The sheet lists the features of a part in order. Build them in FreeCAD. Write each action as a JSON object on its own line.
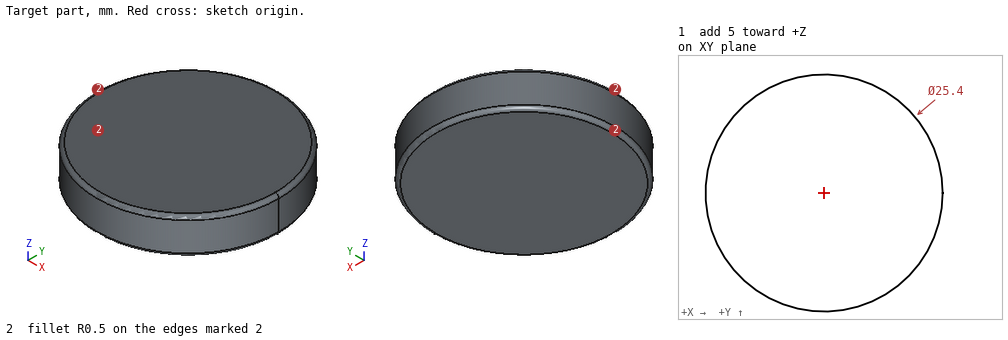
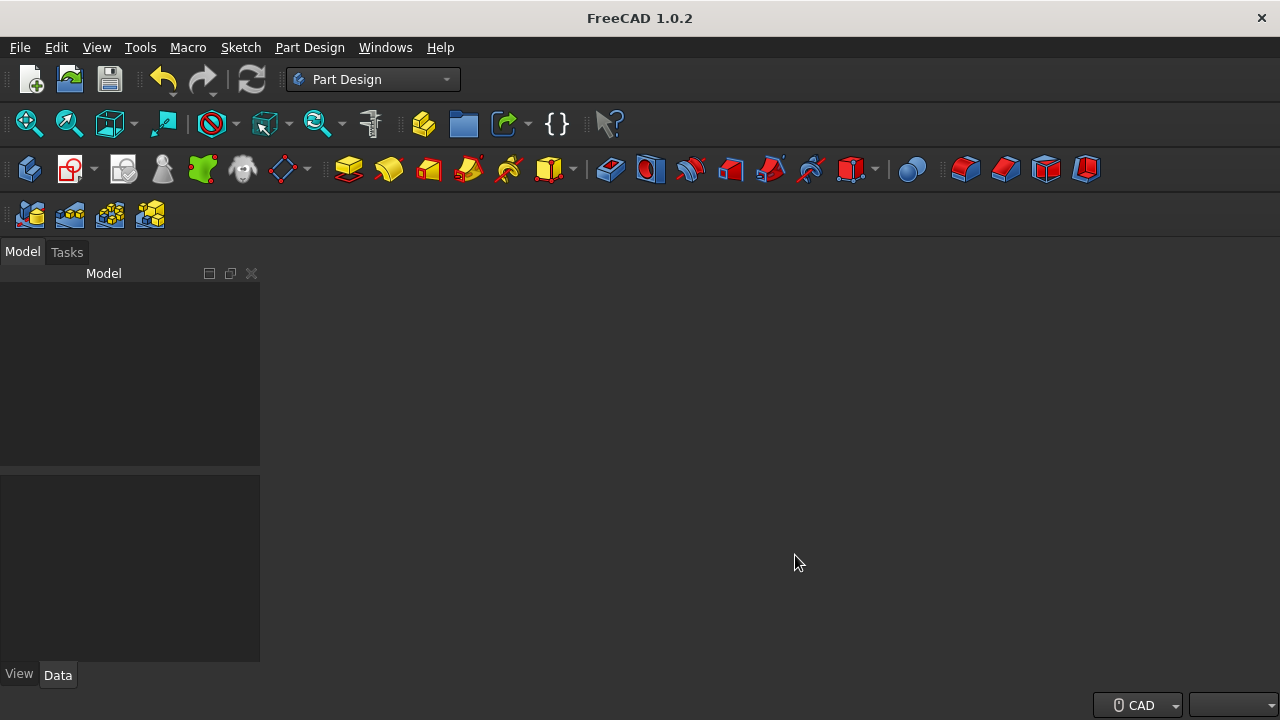
{"action": "left_click", "coordinate": [30, 80]}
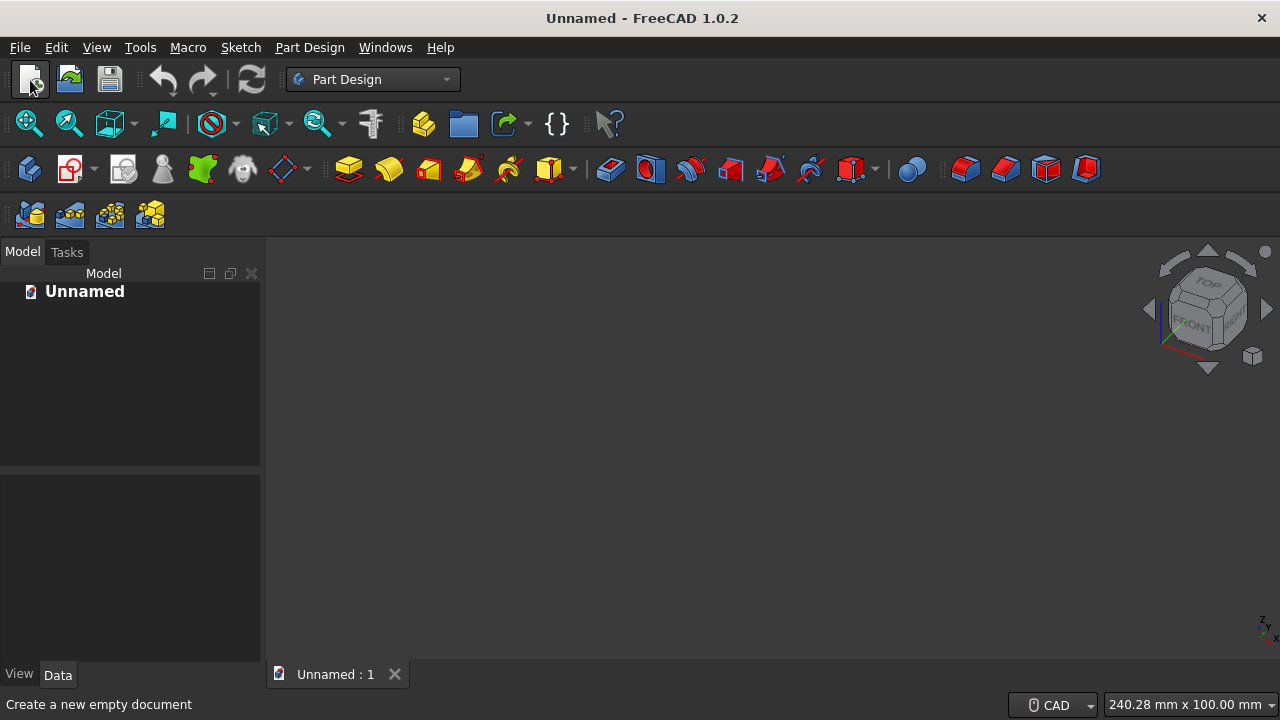
{"action": "left_click", "coordinate": [70, 170]}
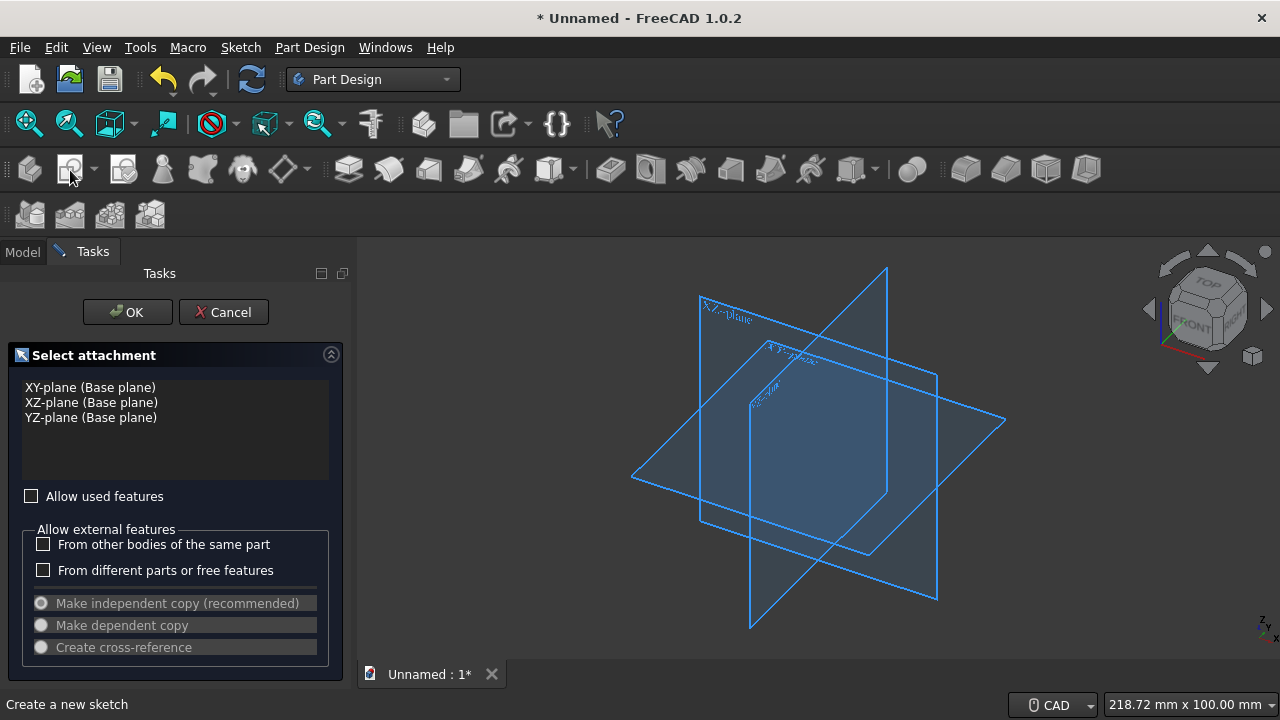
{"action": "left_click", "coordinate": [82, 388]}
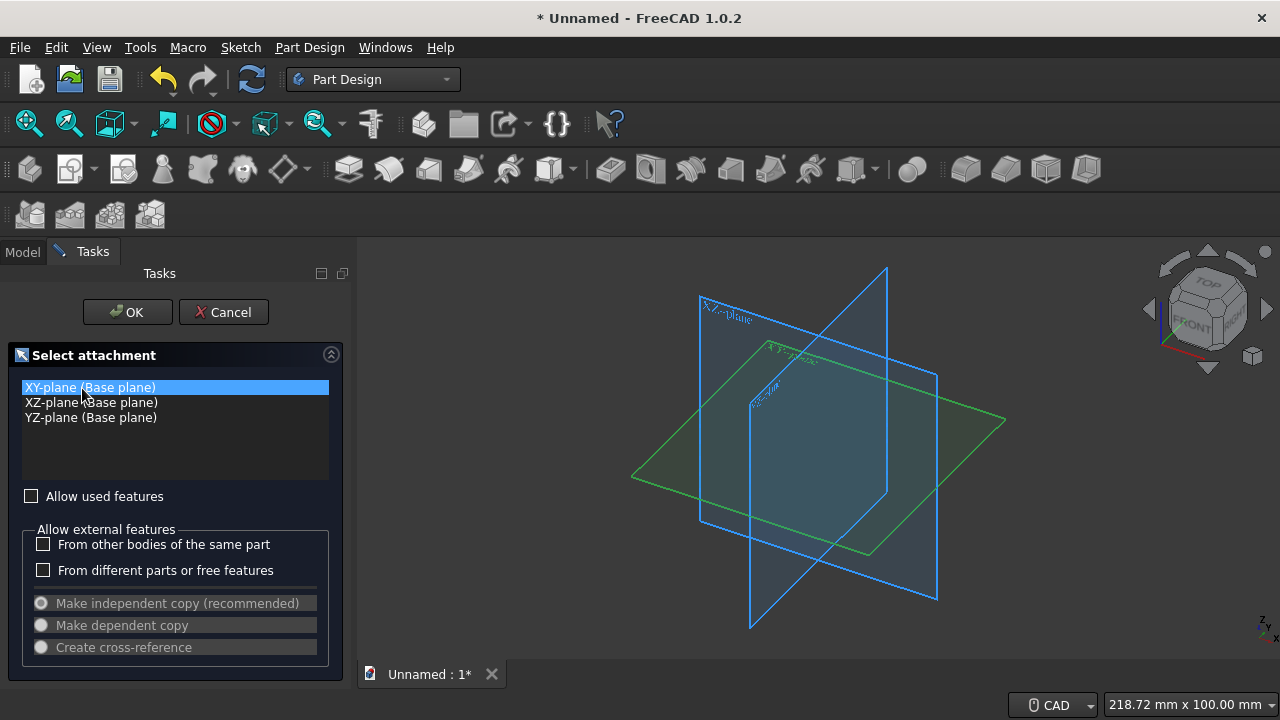
{"action": "left_click", "coordinate": [128, 312]}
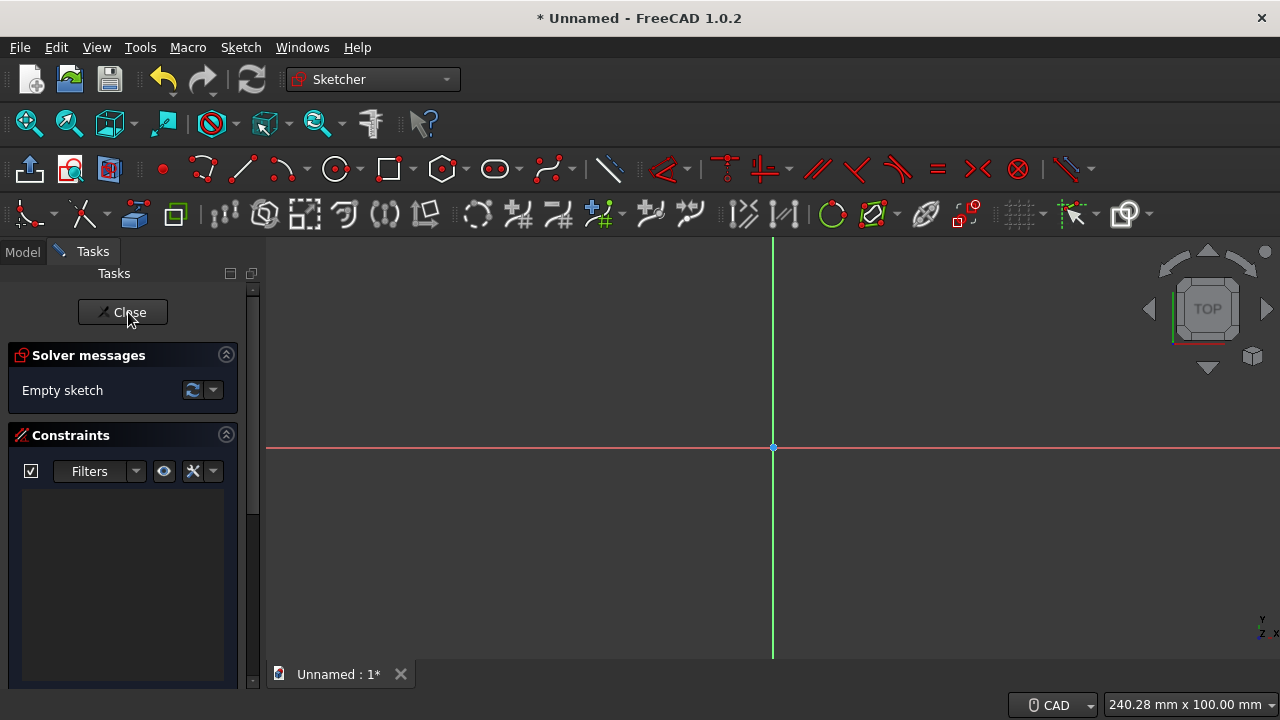
{"action": "scroll", "coordinate": [829, 448], "scroll_direction": "up", "scroll_amount": 4}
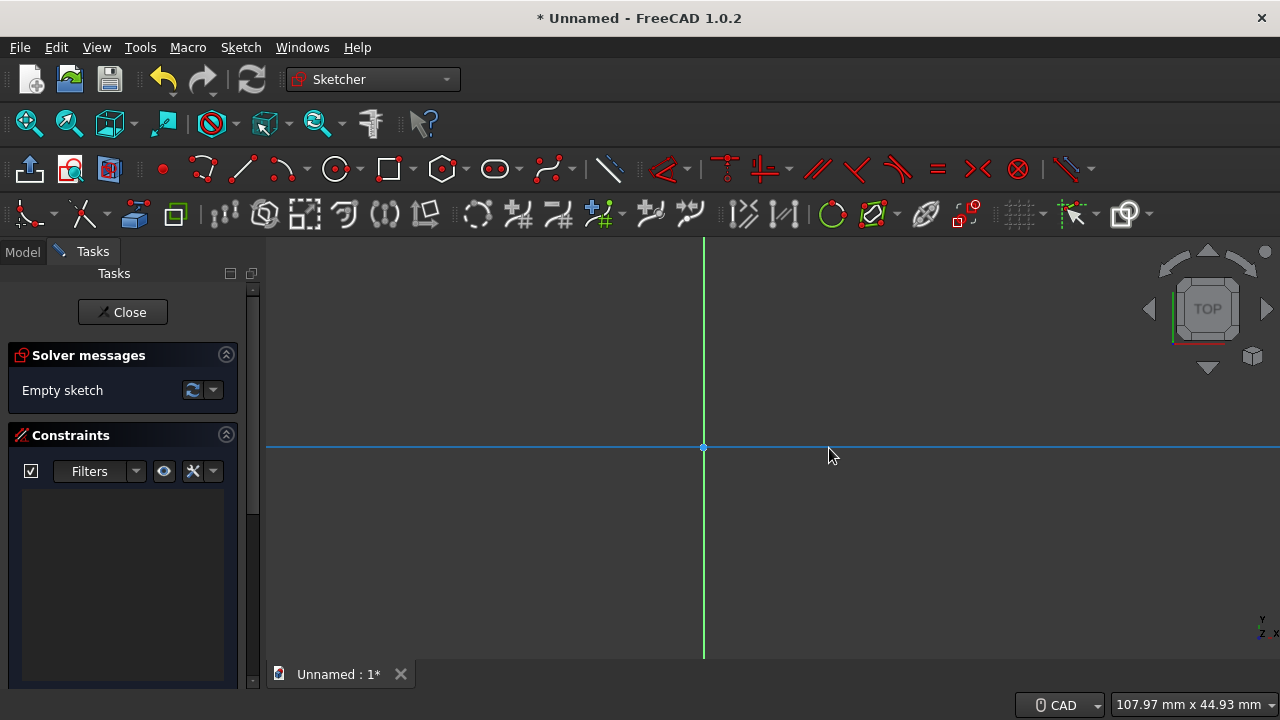
{"action": "left_click", "coordinate": [336, 170]}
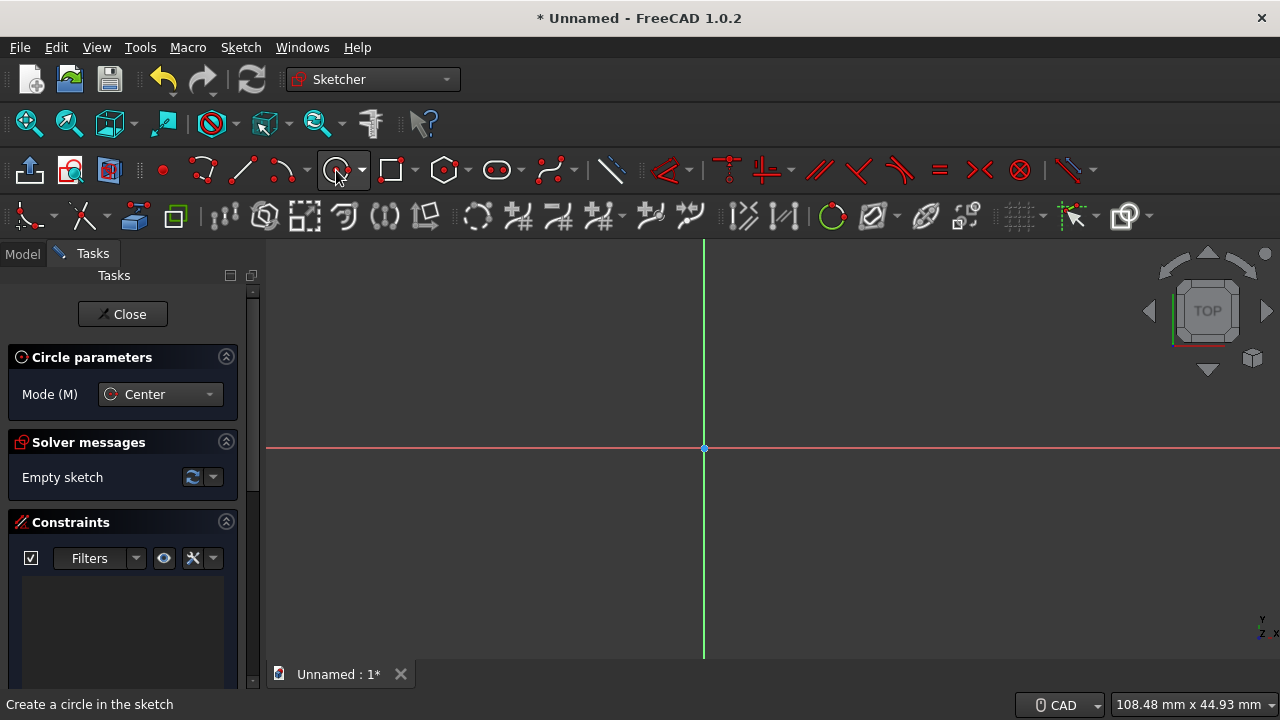
{"action": "left_click", "coordinate": [704, 448]}
{"action": "mouse_move", "coordinate": [788, 364]}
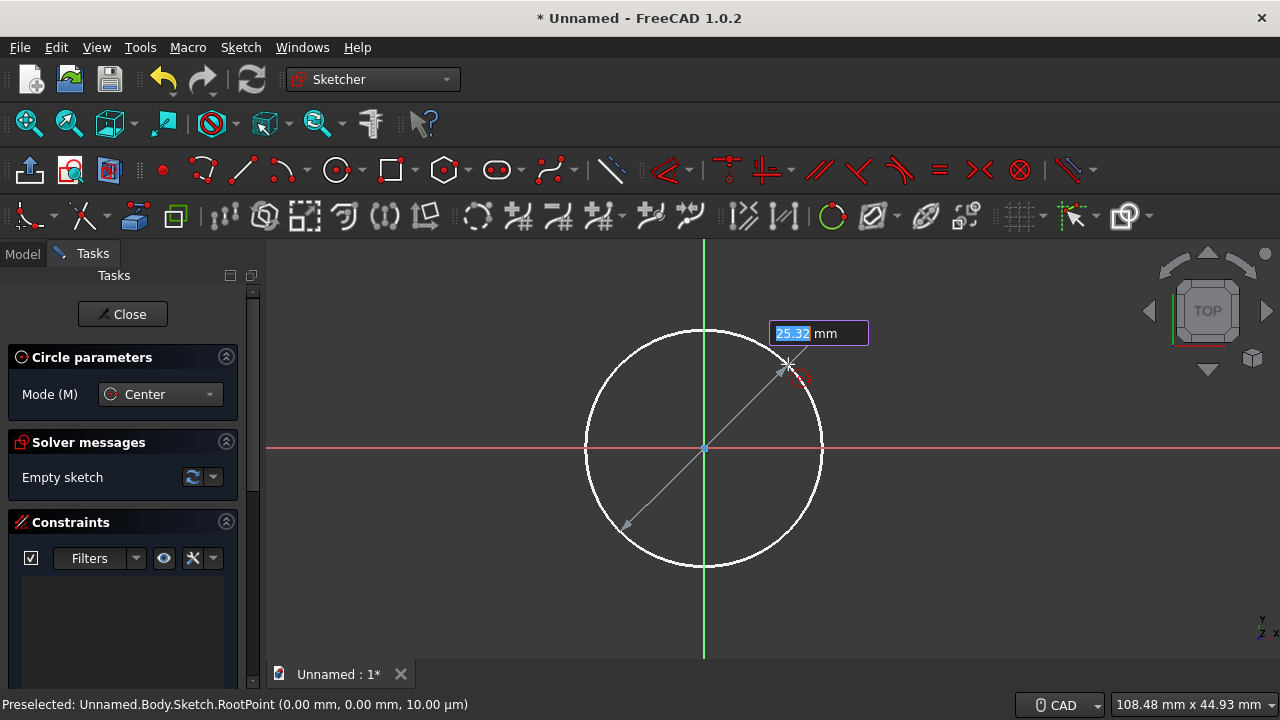
{"action": "type", "text": "25.4"}
{"action": "key", "text": "Return"}
{"action": "key", "text": "Escape"}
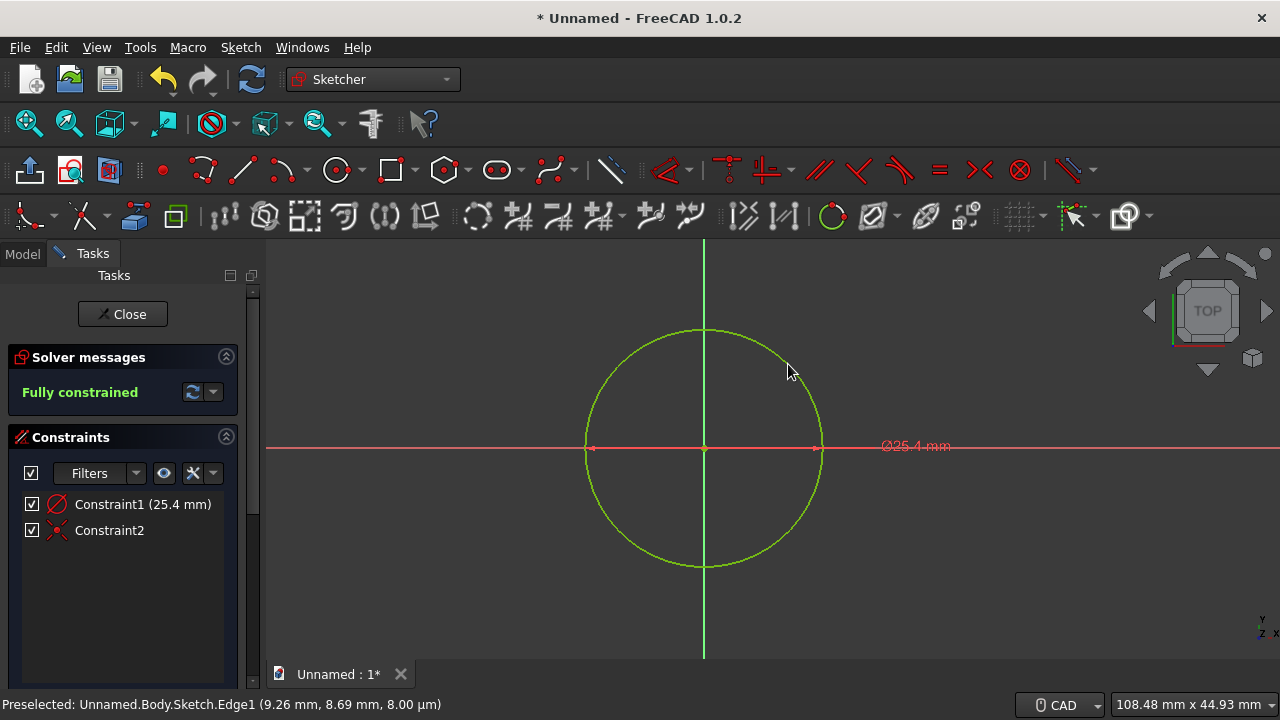
{"action": "left_click", "coordinate": [123, 314]}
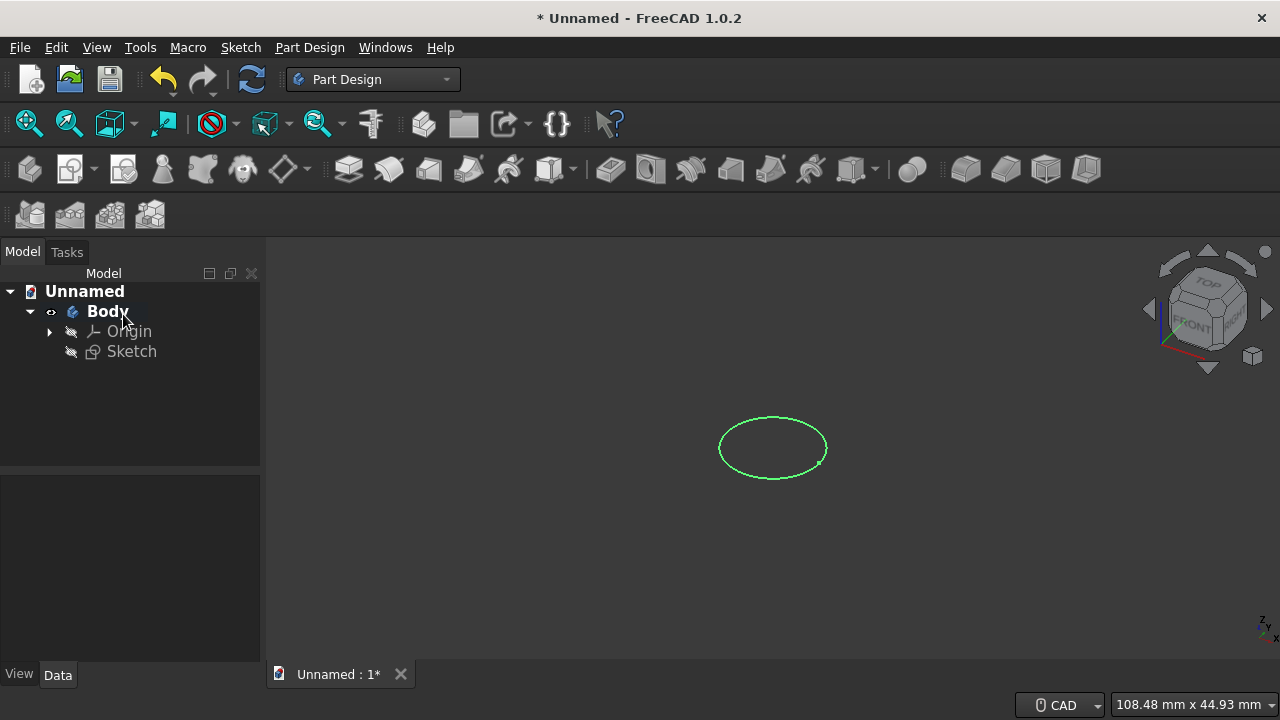
{"action": "left_click", "coordinate": [350, 170]}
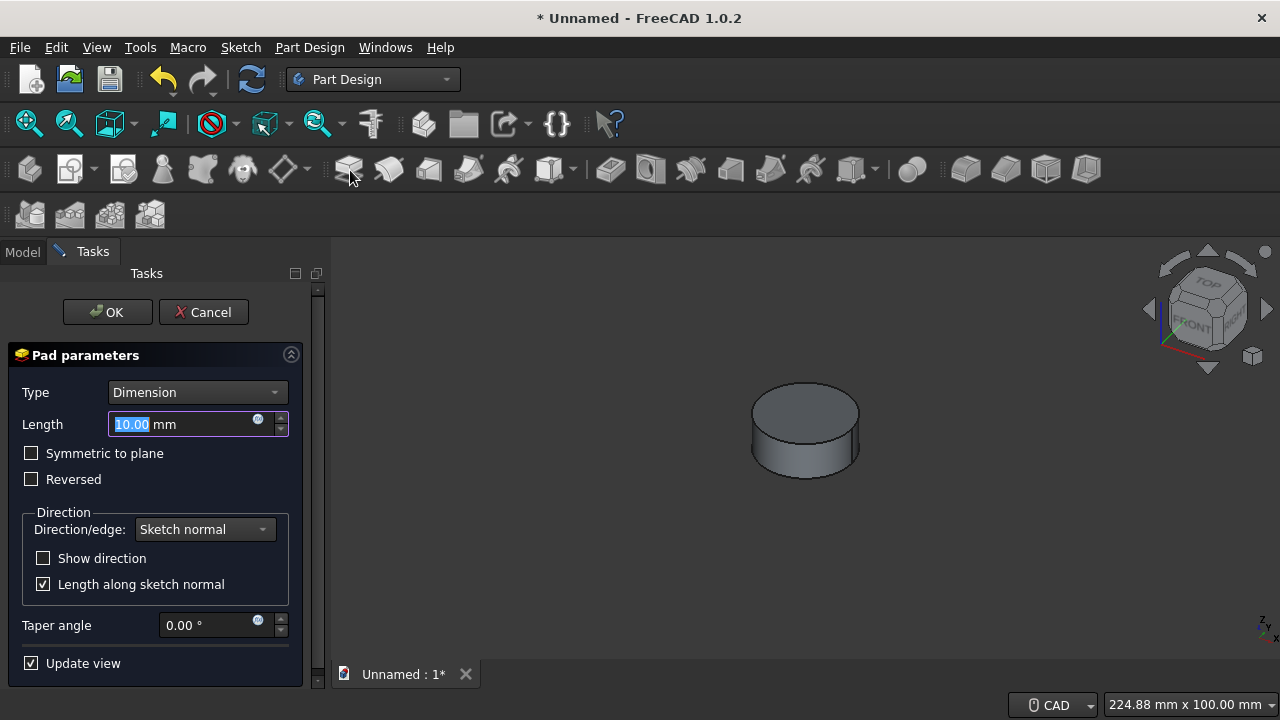
{"action": "type", "text": "5"}
{"action": "key", "text": "Tab"}